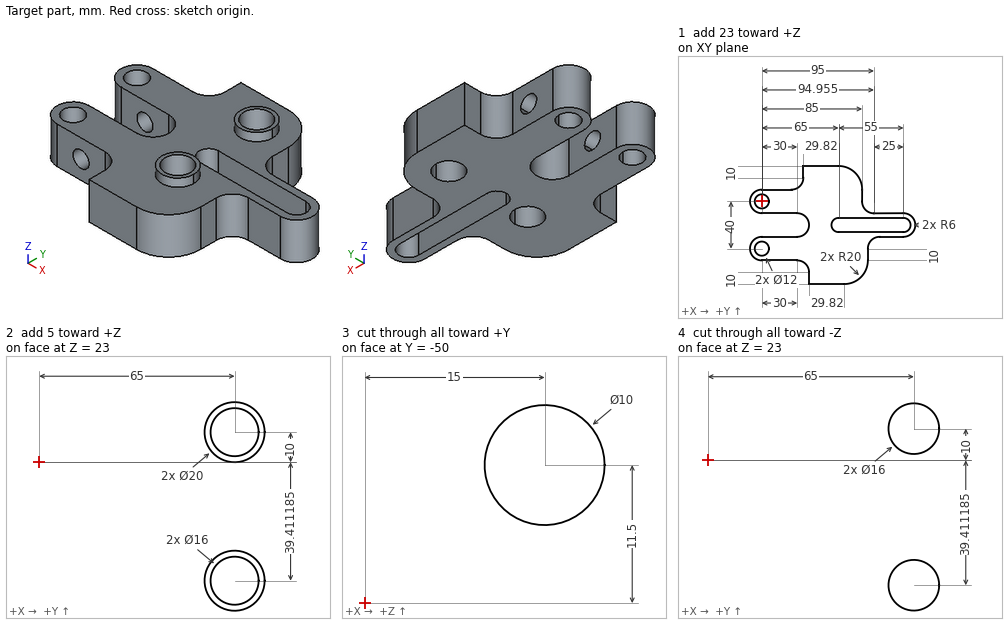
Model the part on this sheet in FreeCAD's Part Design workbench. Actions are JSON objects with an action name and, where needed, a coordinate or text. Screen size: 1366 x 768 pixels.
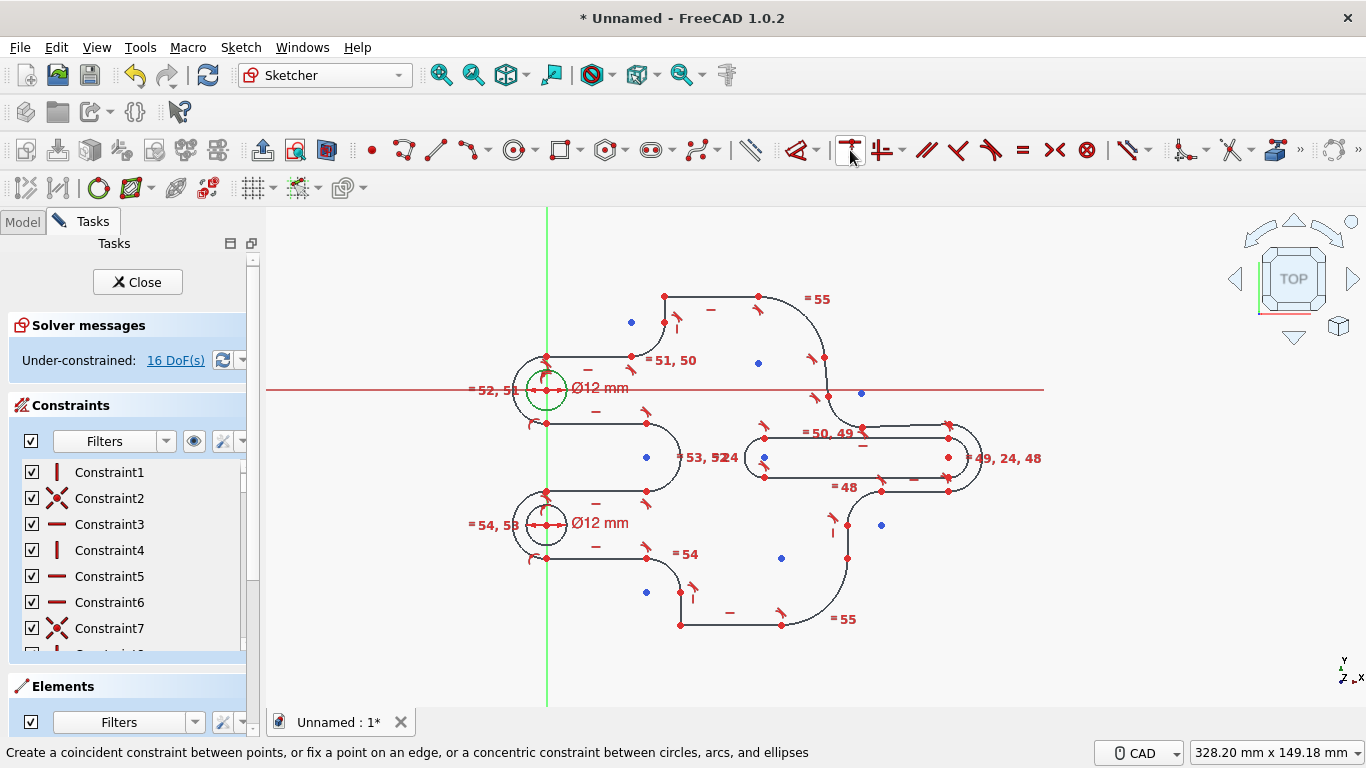
{"action": "key", "text": "d"}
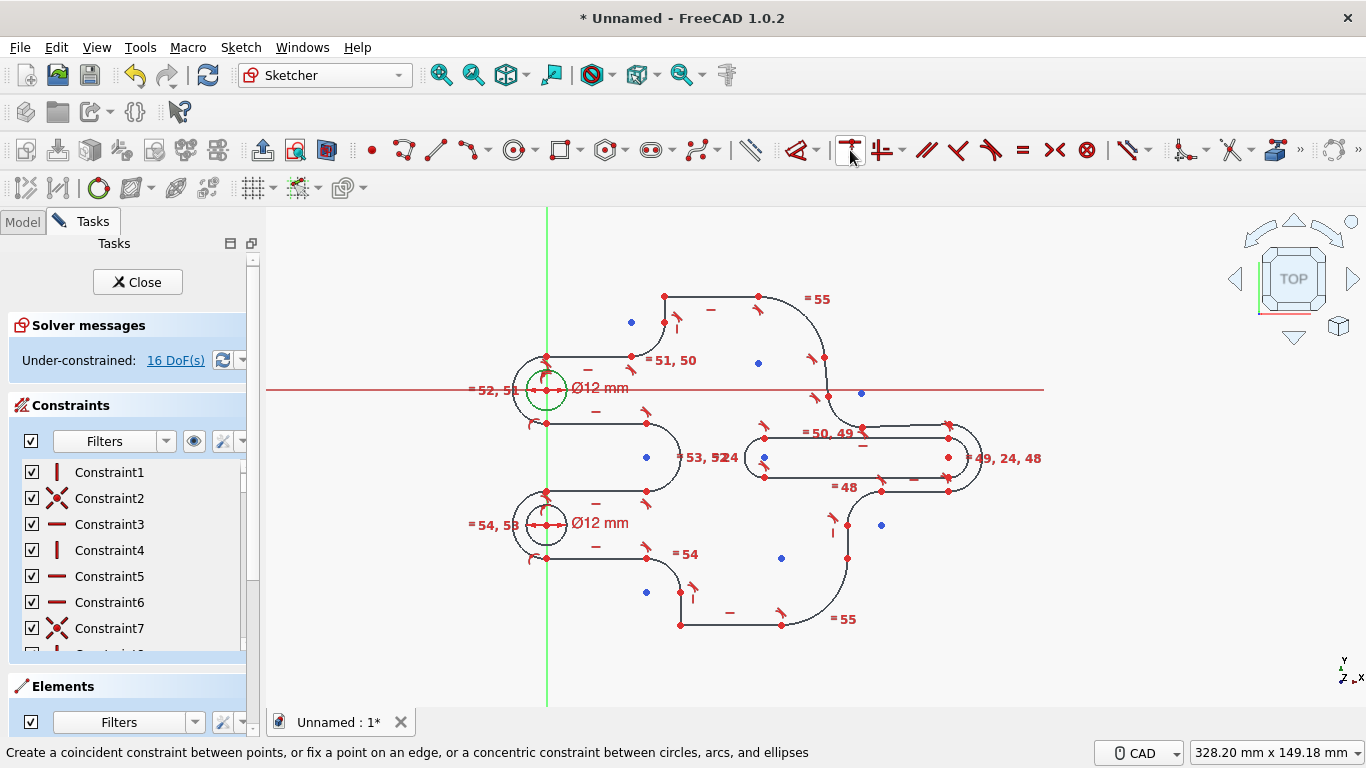
{"action": "left_click", "coordinate": [811, 618]}
{"action": "left_click", "coordinate": [825, 647]}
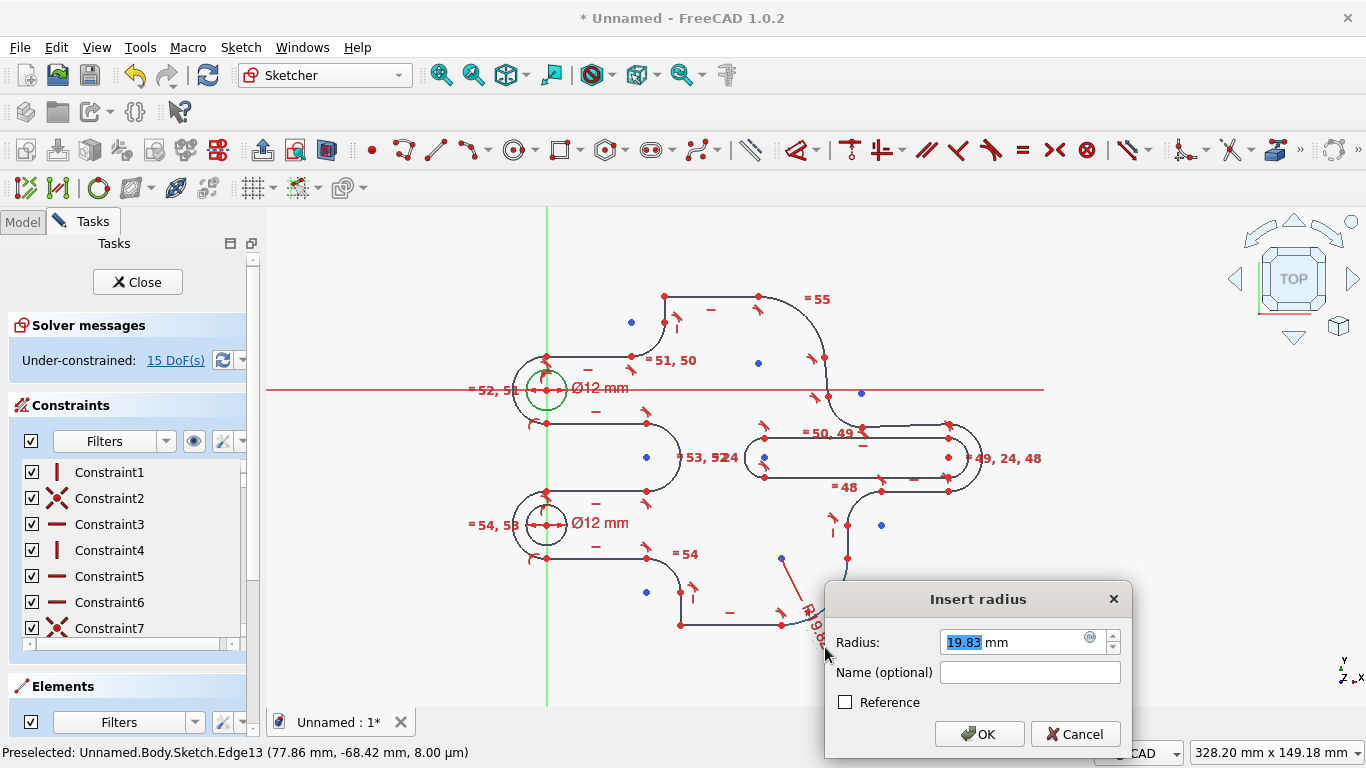
{"action": "type", "text": "20"}
{"action": "key", "text": "Return"}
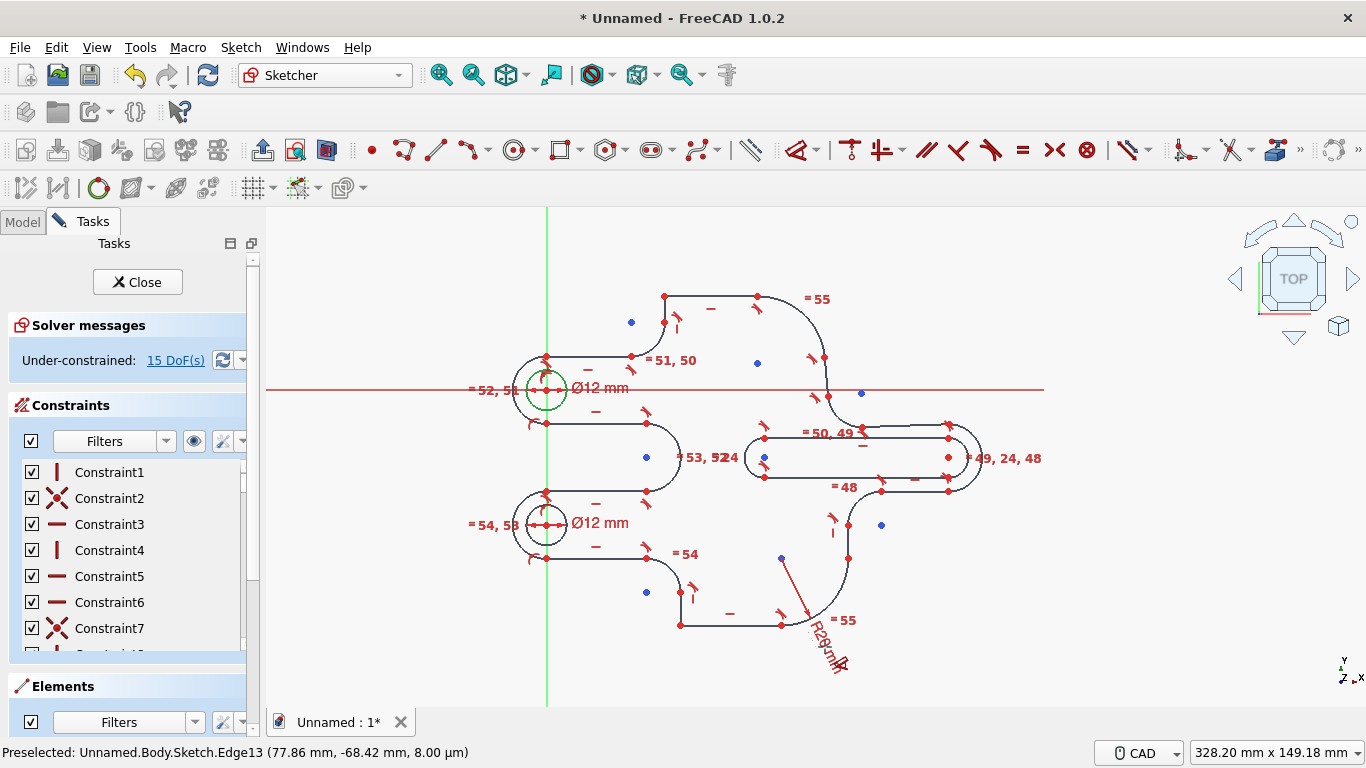
{"action": "scroll", "coordinate": [748, 446], "scroll_direction": "up", "scroll_amount": 4}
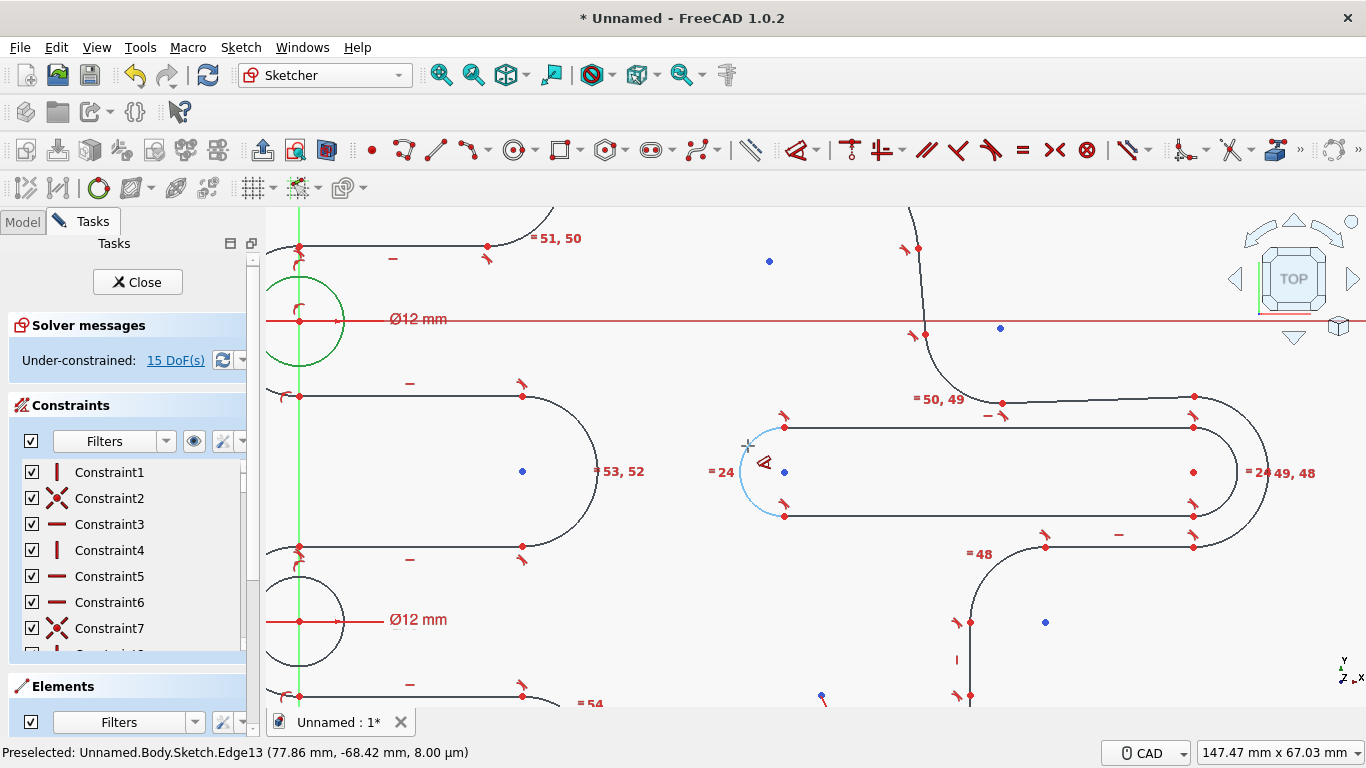
{"action": "left_click", "coordinate": [749, 446]}
{"action": "left_click", "coordinate": [723, 427]}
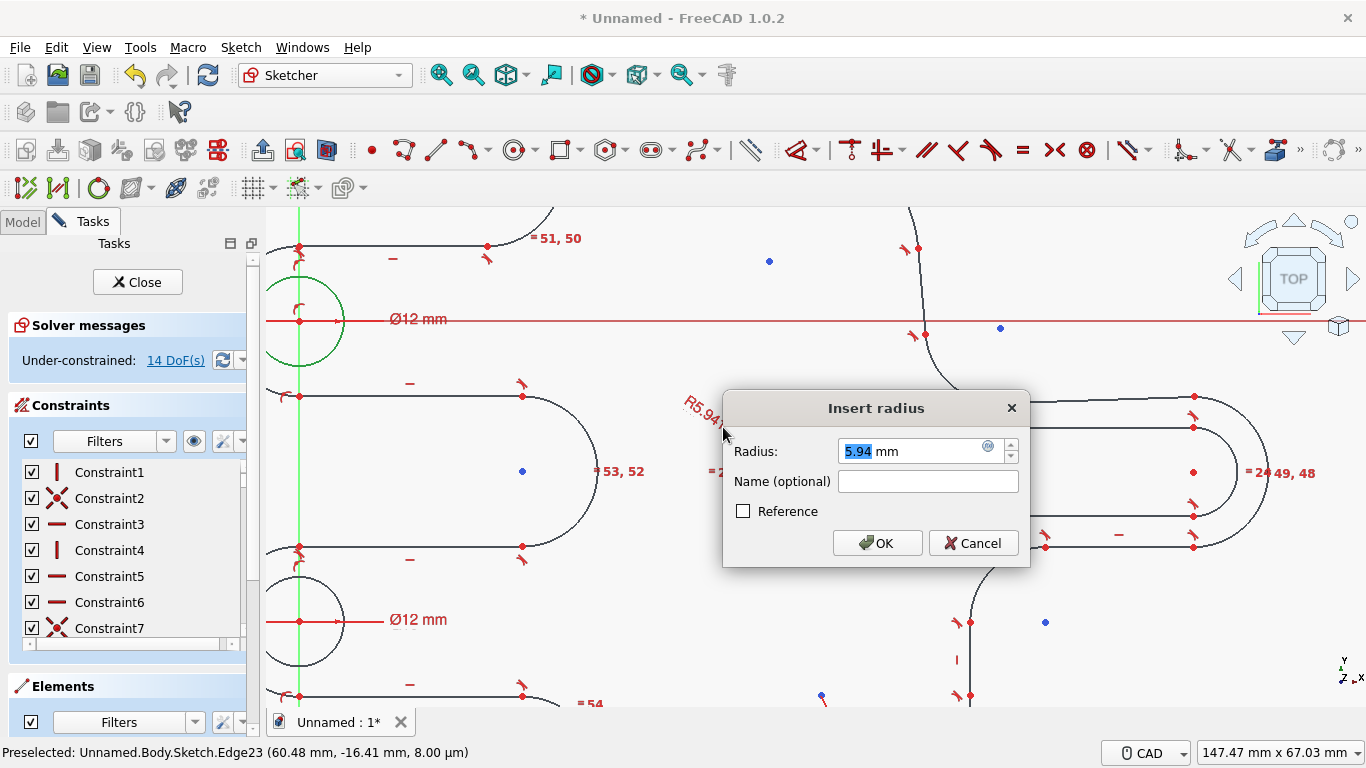
{"action": "type", "text": "6"}
{"action": "key", "text": "Return"}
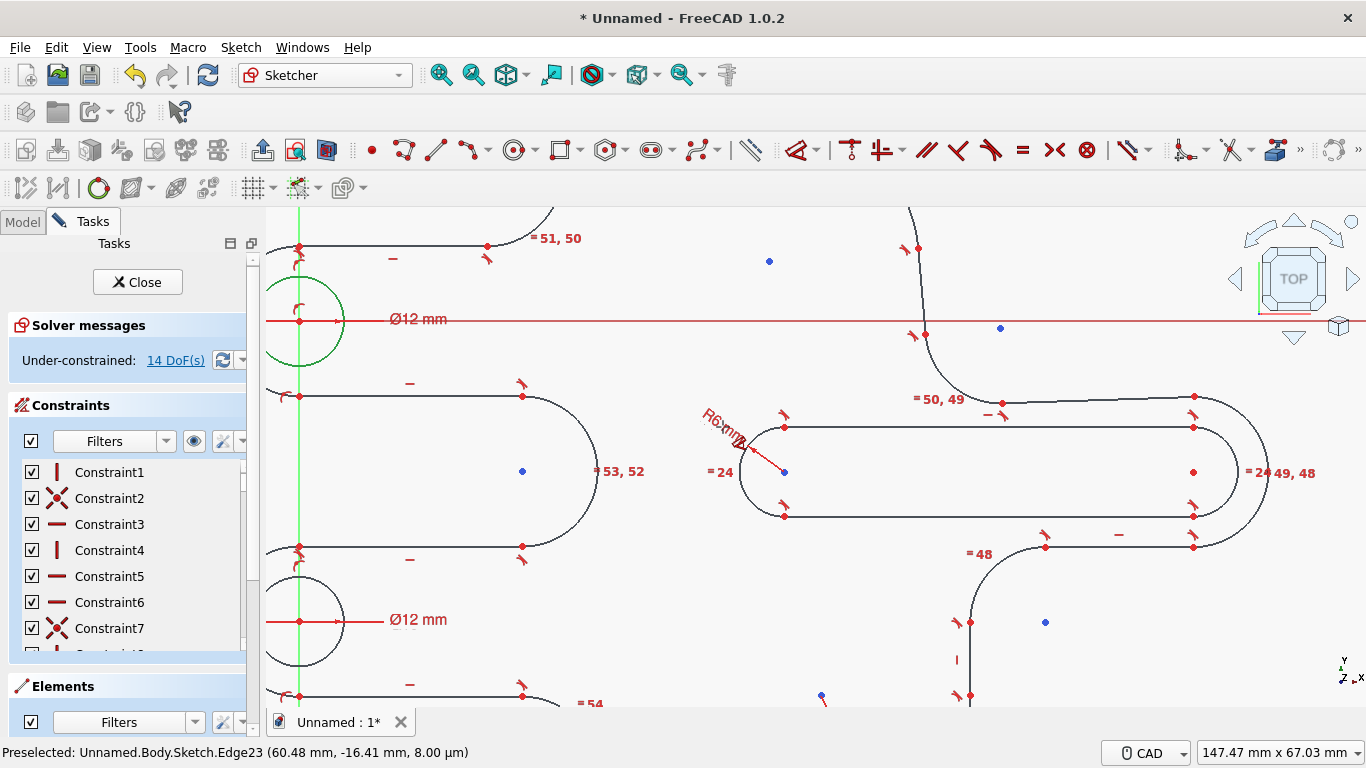
{"action": "scroll", "coordinate": [748, 446], "scroll_direction": "down", "scroll_amount": 4}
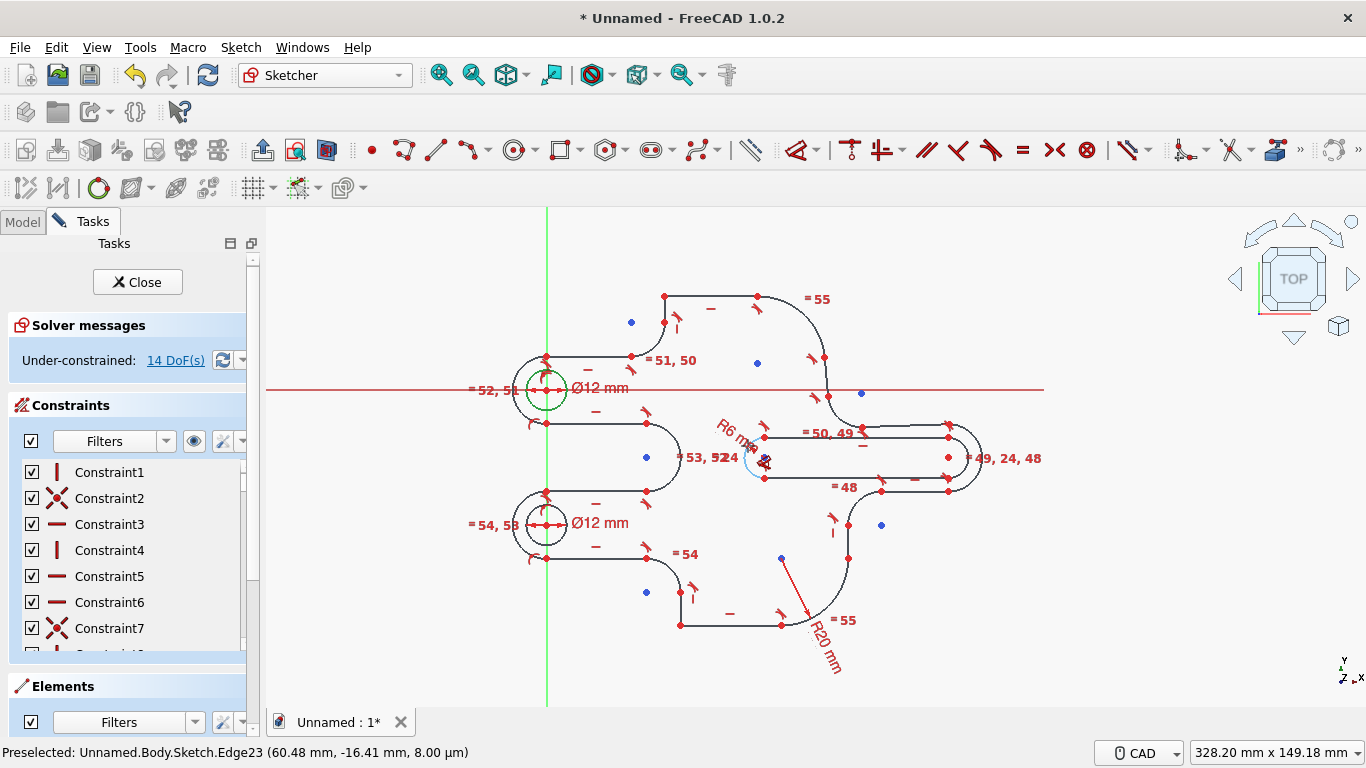
{"action": "scroll", "coordinate": [681, 603], "scroll_direction": "up", "scroll_amount": 2}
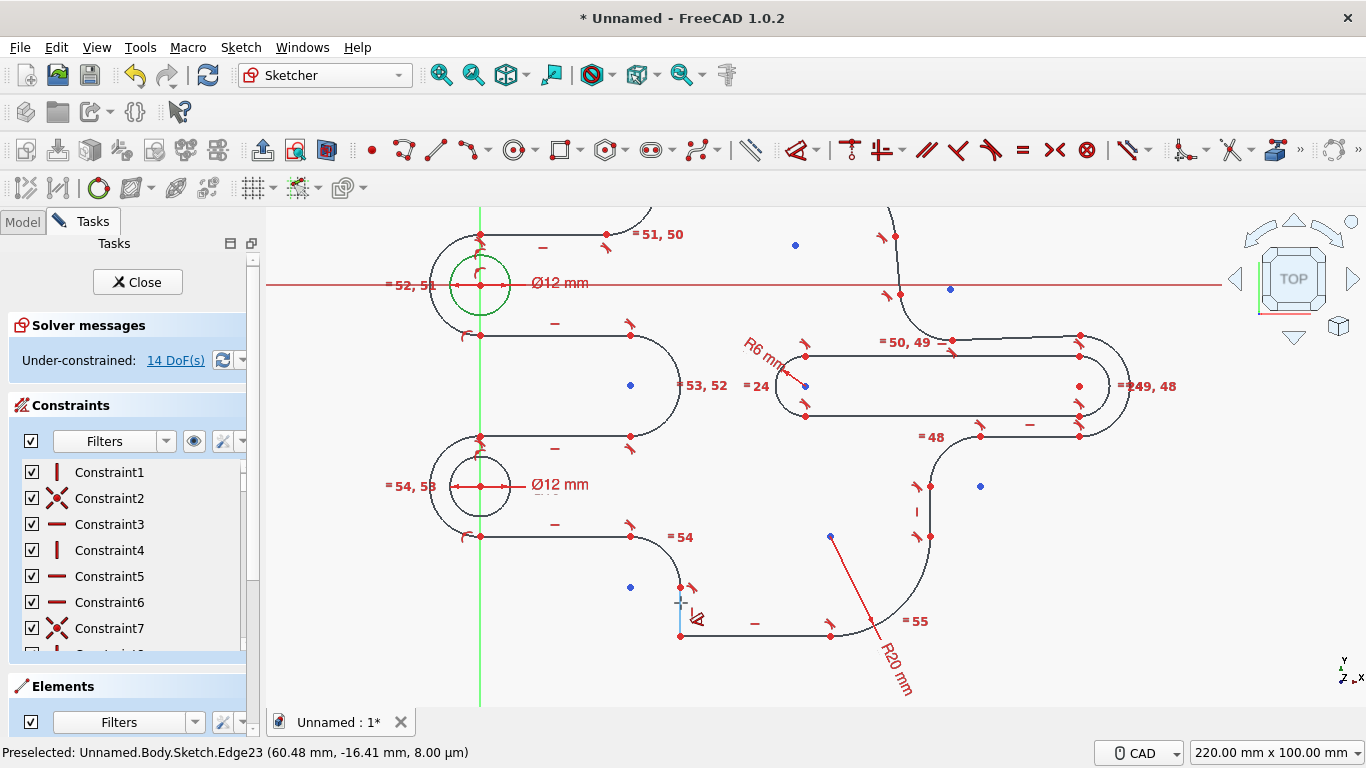
{"action": "left_click", "coordinate": [680, 602]}
{"action": "left_click", "coordinate": [646, 612]}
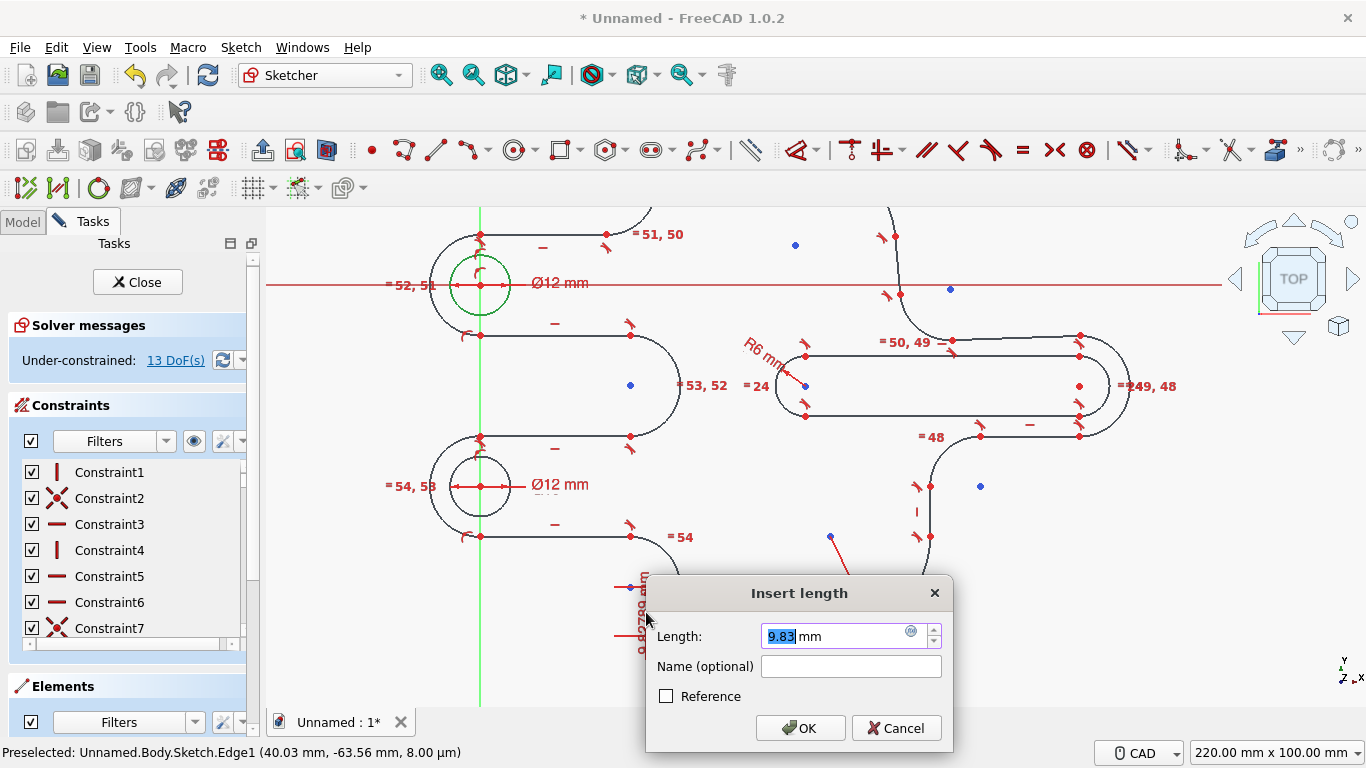
{"action": "type", "text": "10"}
{"action": "key", "text": "Return"}